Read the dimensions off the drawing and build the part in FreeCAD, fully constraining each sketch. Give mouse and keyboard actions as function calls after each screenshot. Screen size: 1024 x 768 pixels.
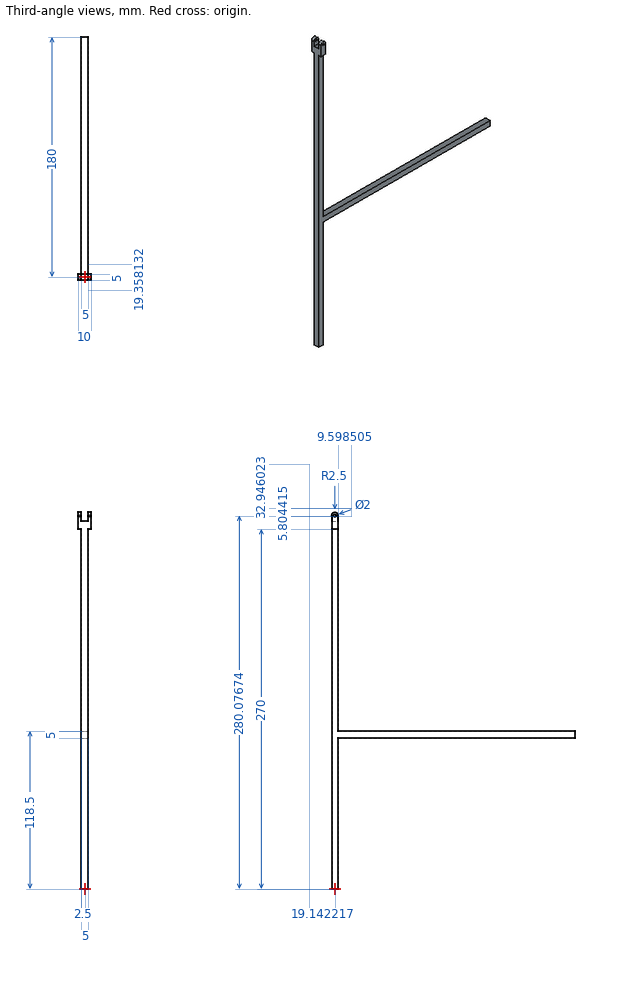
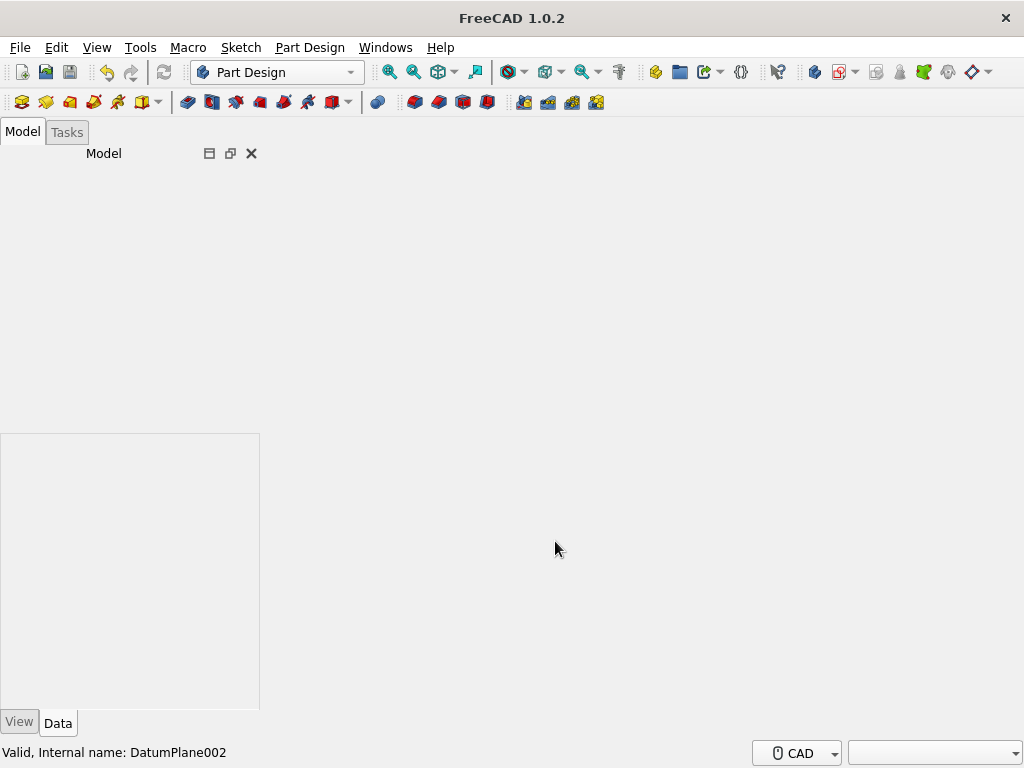
click(22, 72)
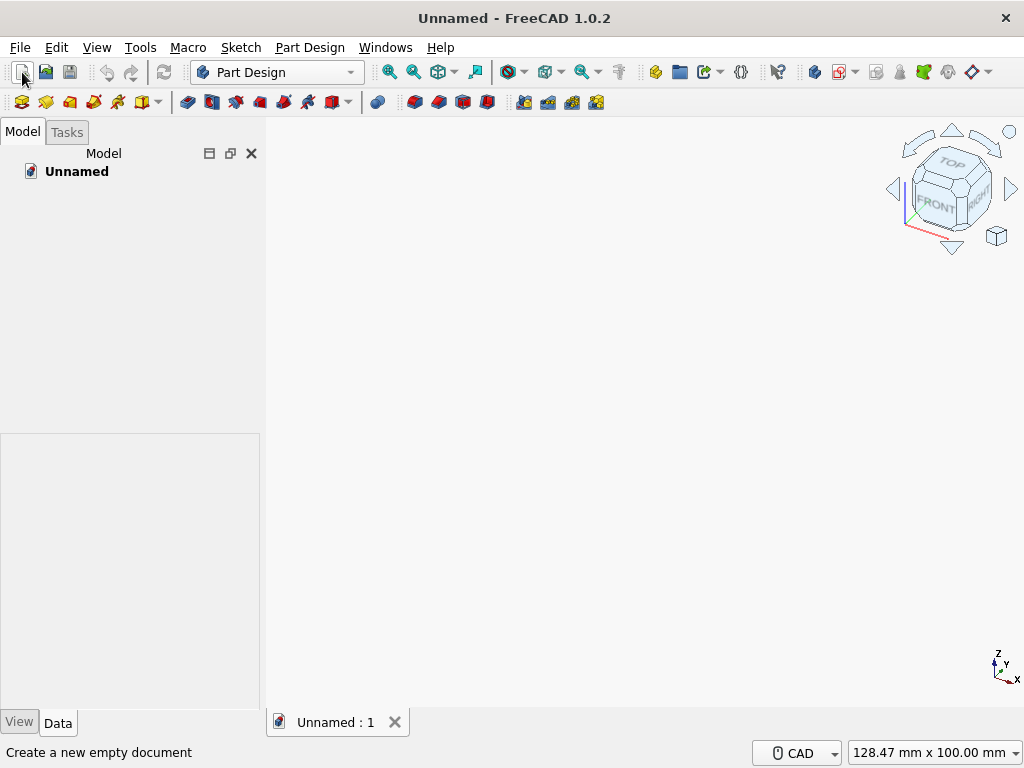
click(840, 72)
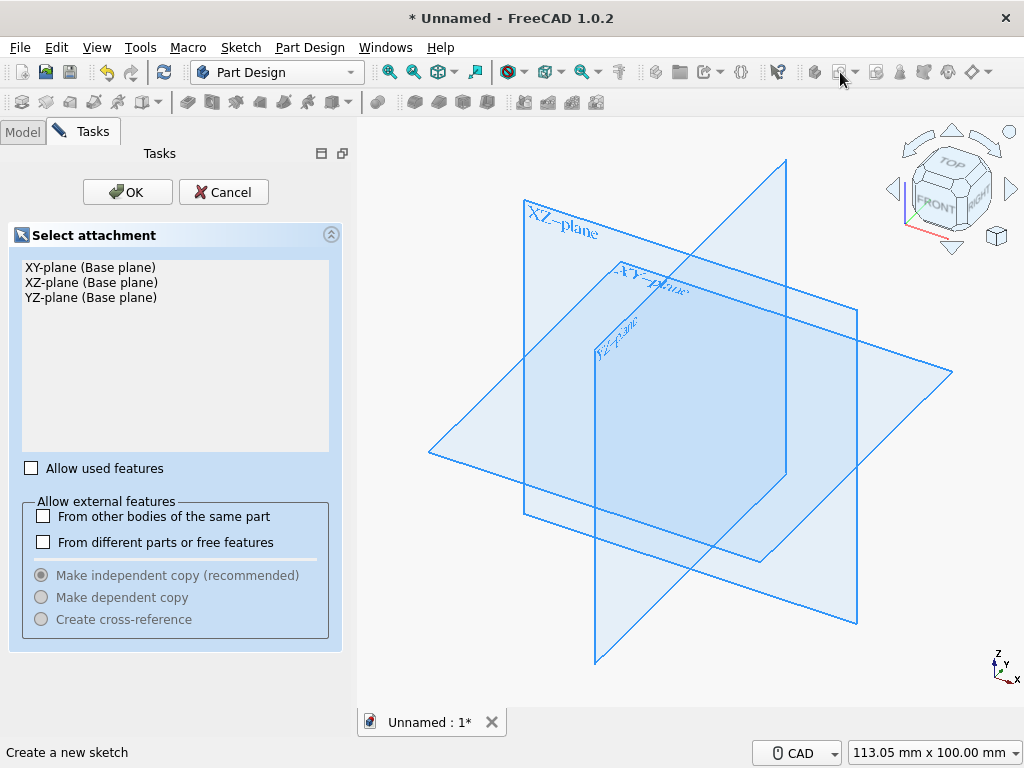
click(82, 268)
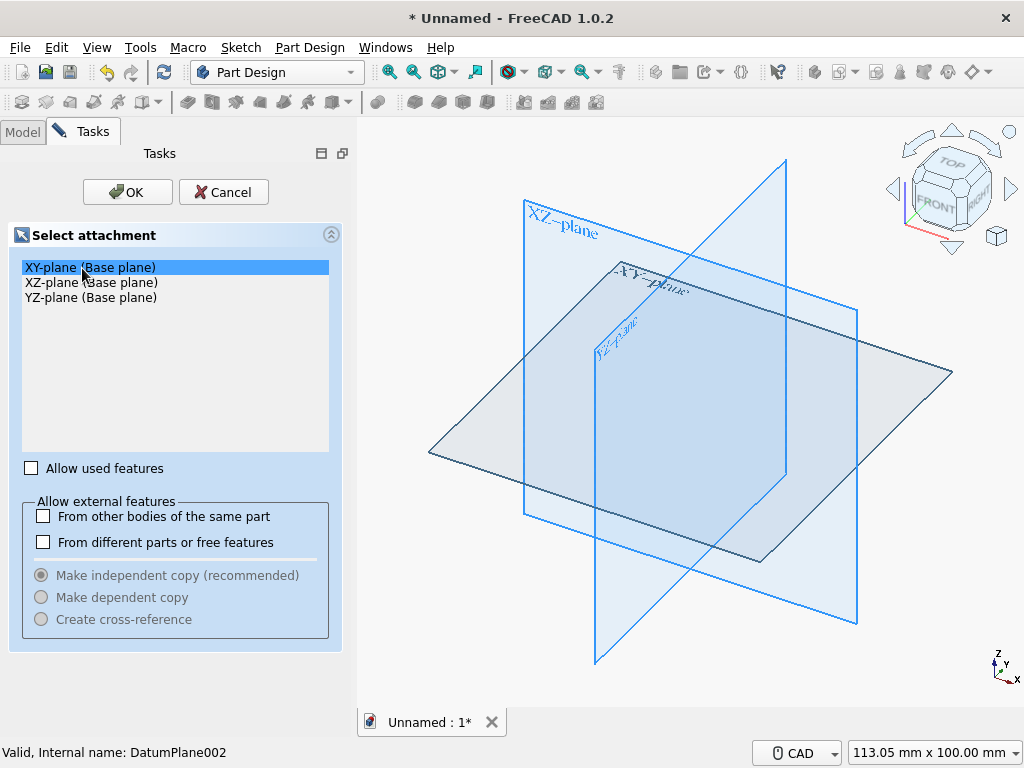
click(128, 192)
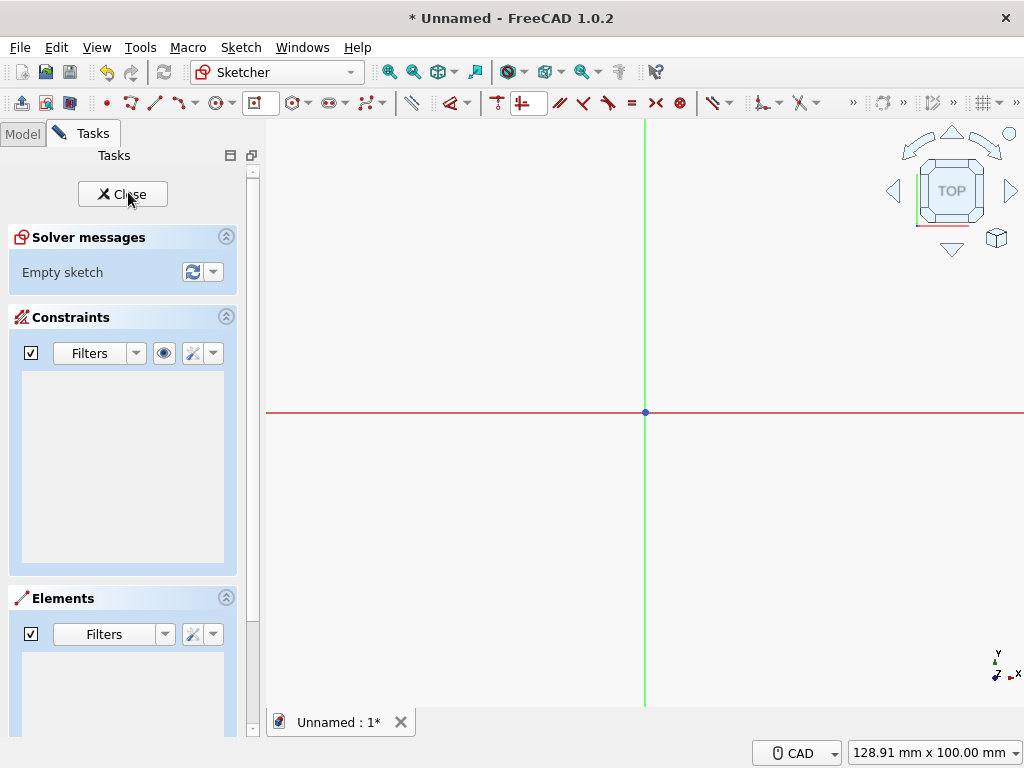
scroll(650, 413, up, 13)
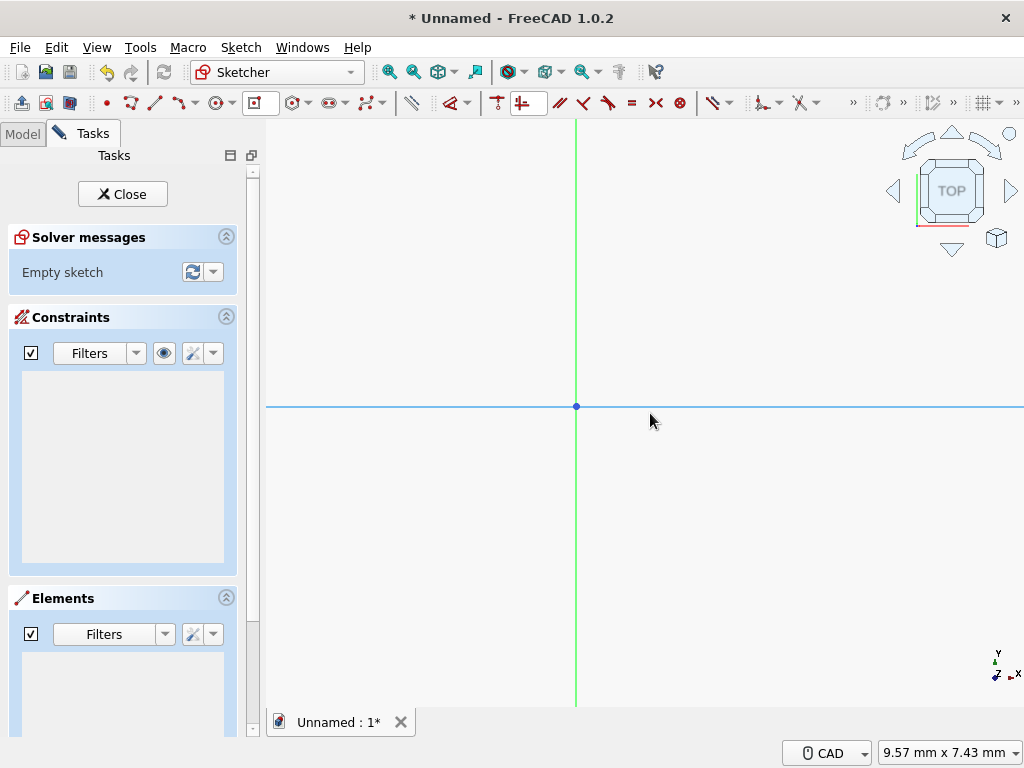
click(254, 104)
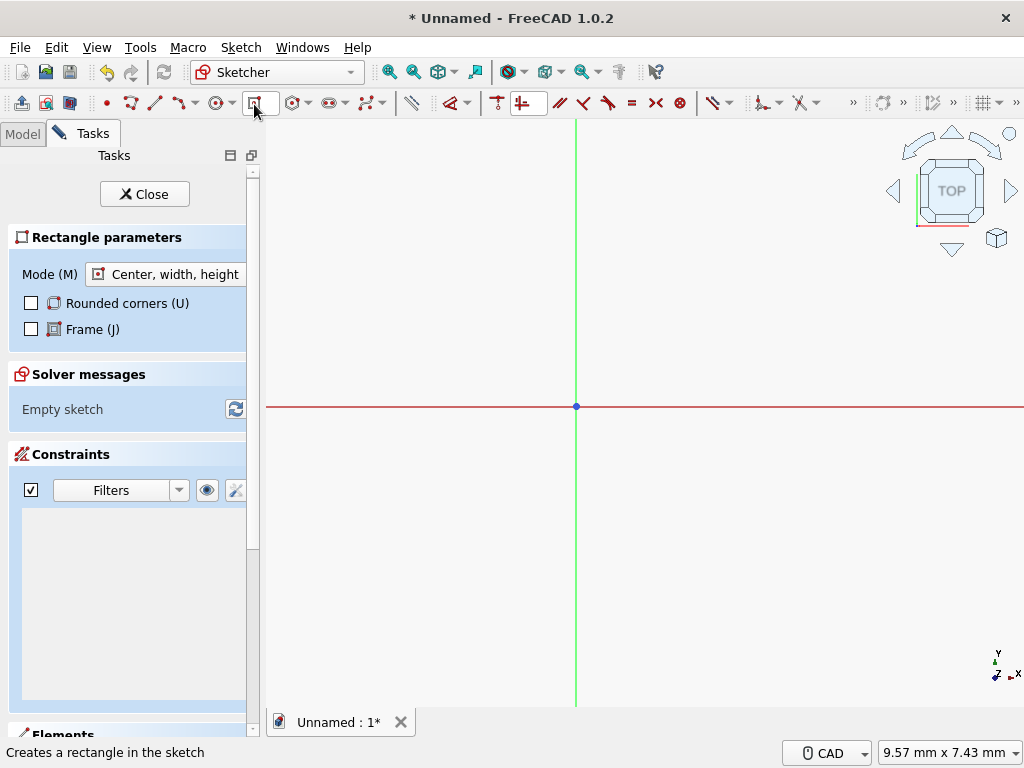
click(576, 407)
click(774, 209)
key(Escape)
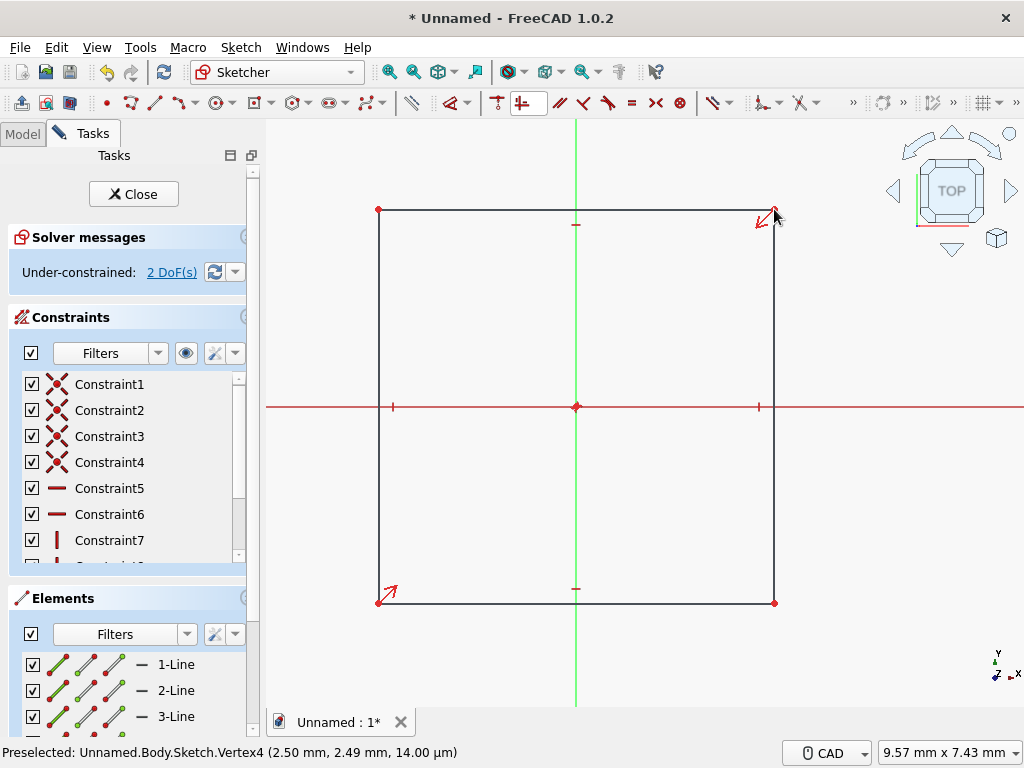
click(450, 104)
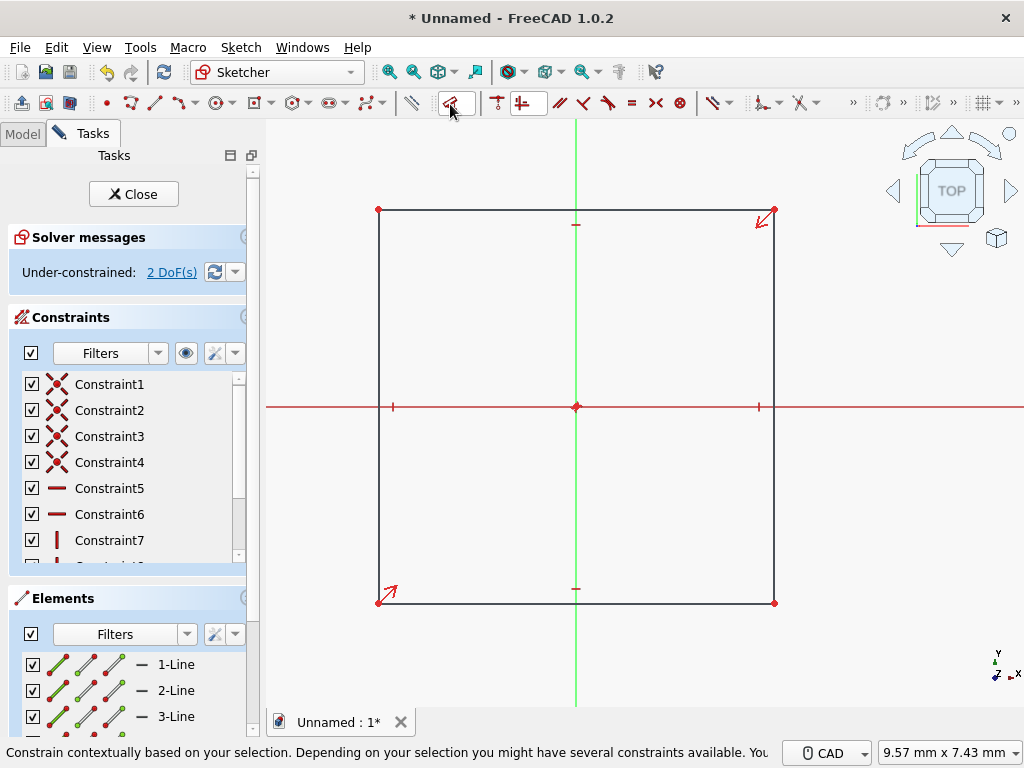
click(497, 604)
click(485, 638)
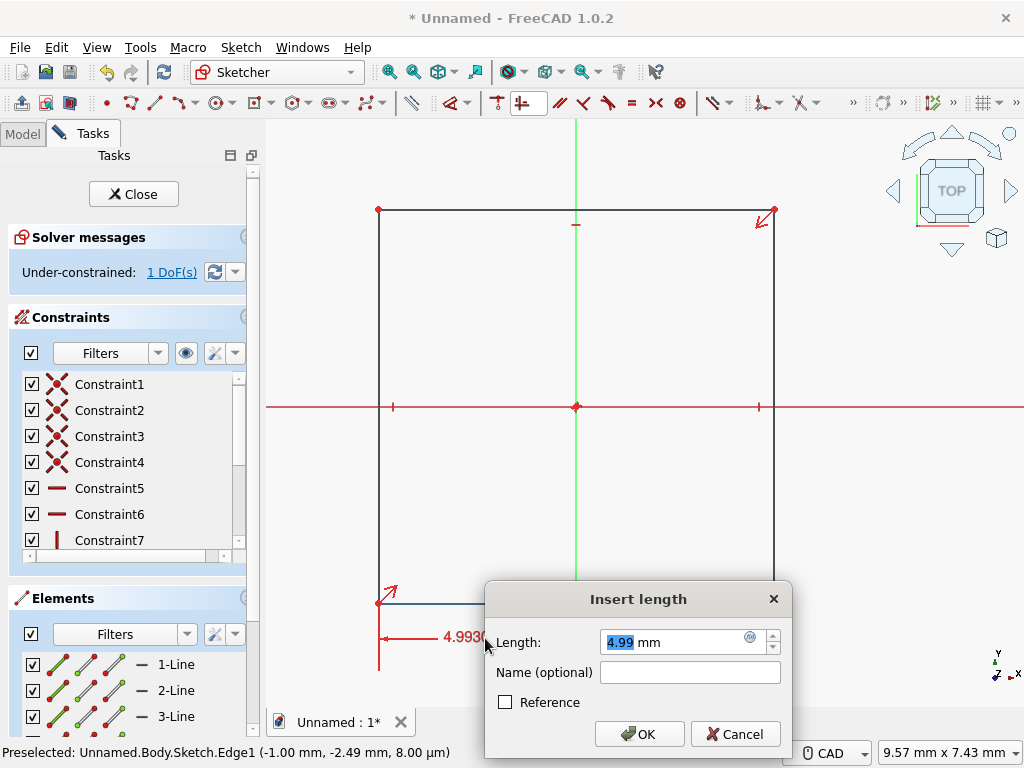
text(5)
key(Return)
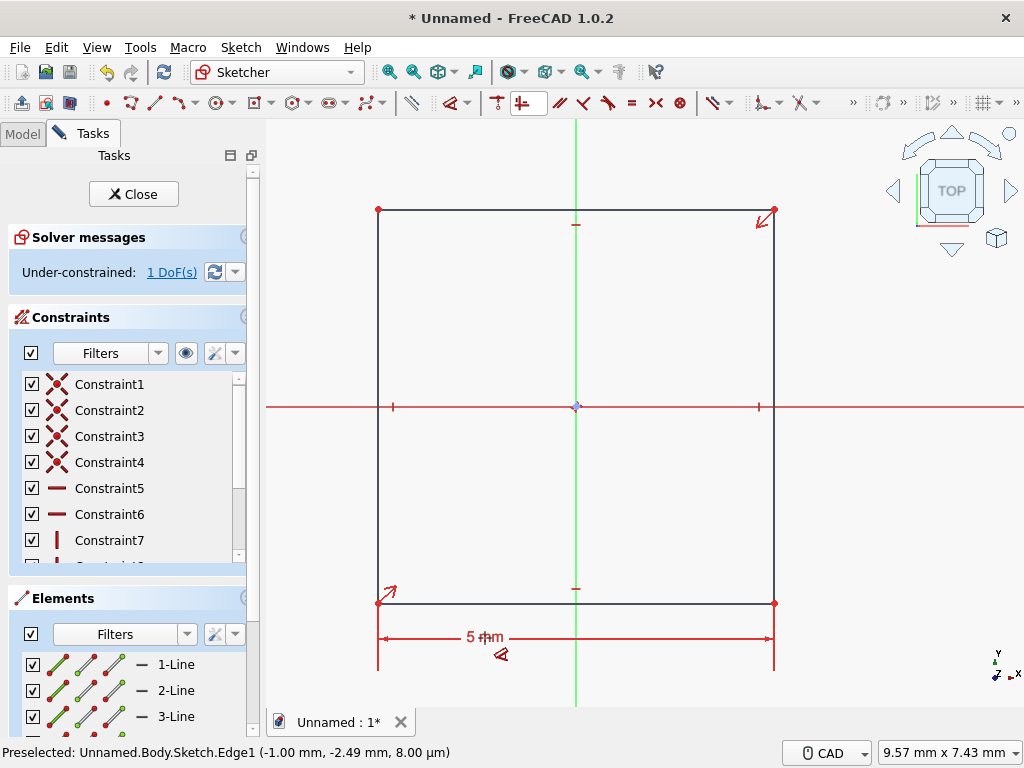
click(774, 485)
click(808, 316)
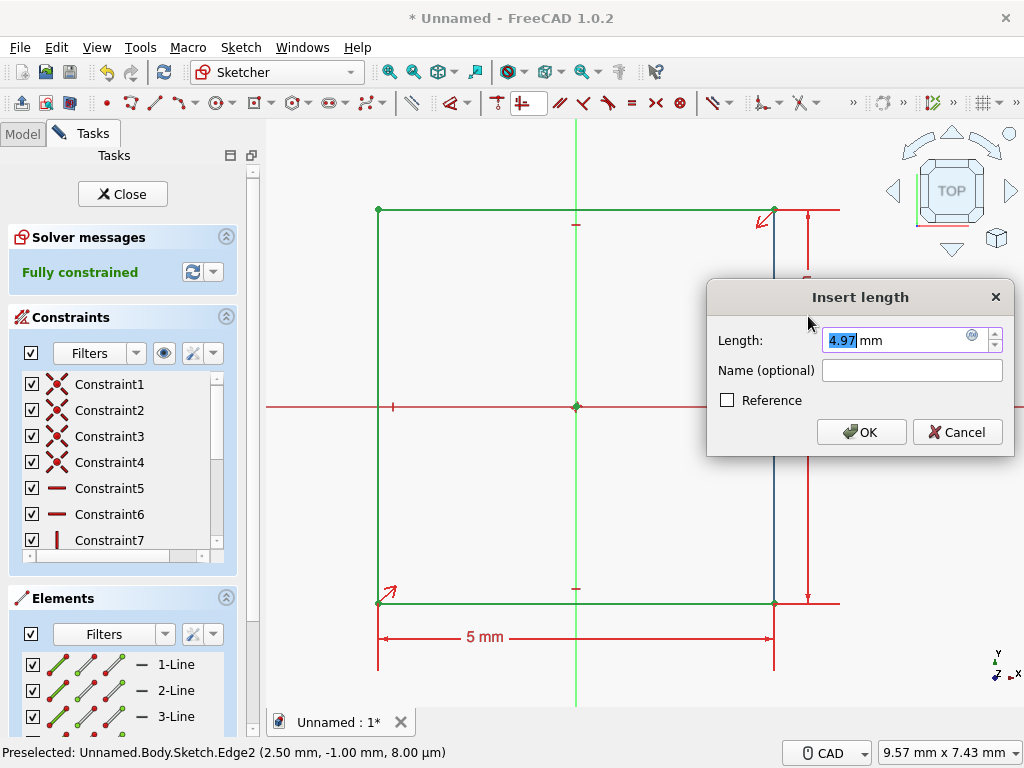
text(5)
key(Return)
key(Escape)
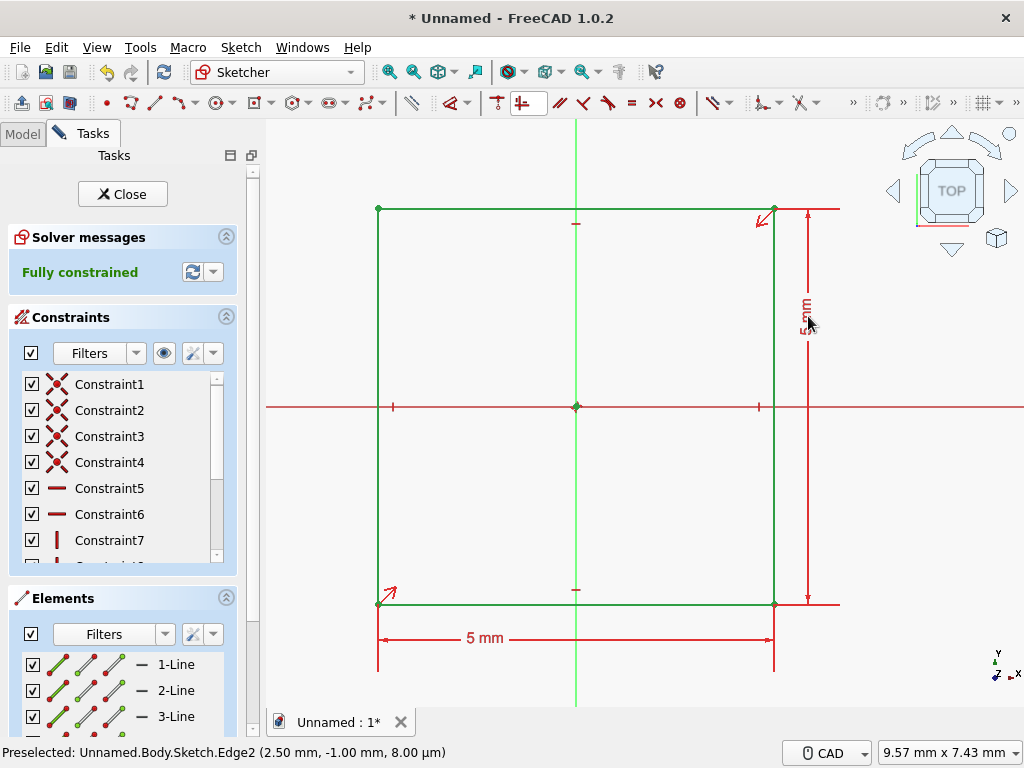
click(123, 194)